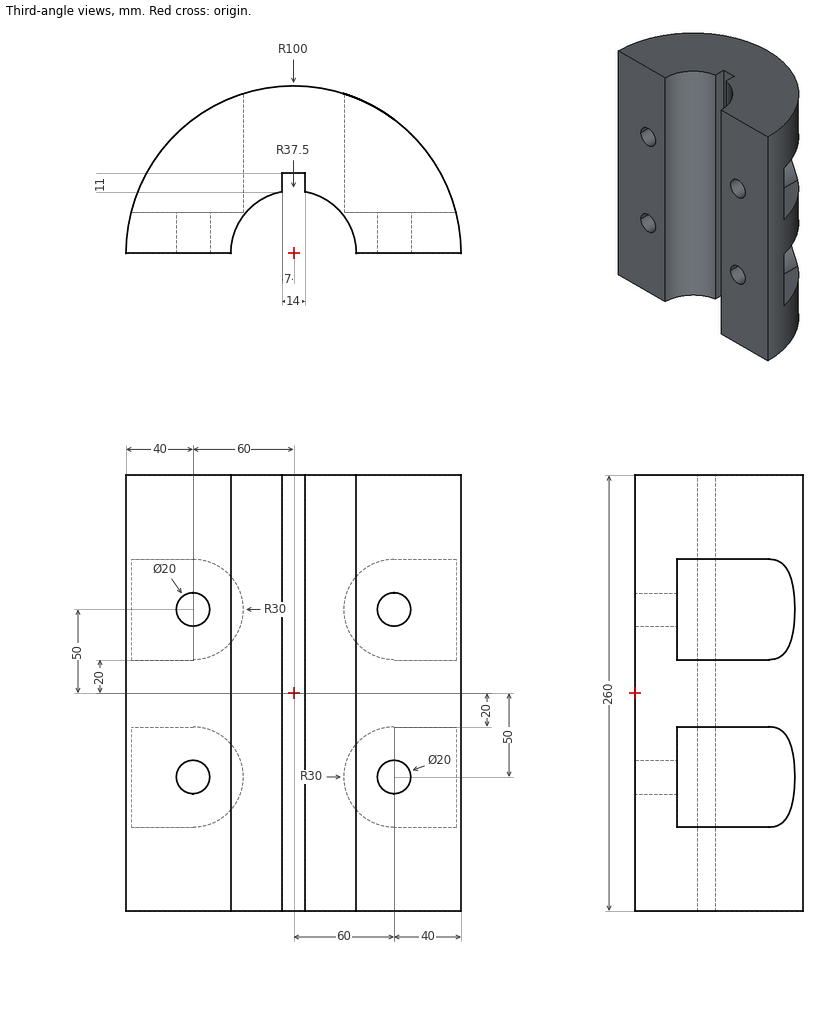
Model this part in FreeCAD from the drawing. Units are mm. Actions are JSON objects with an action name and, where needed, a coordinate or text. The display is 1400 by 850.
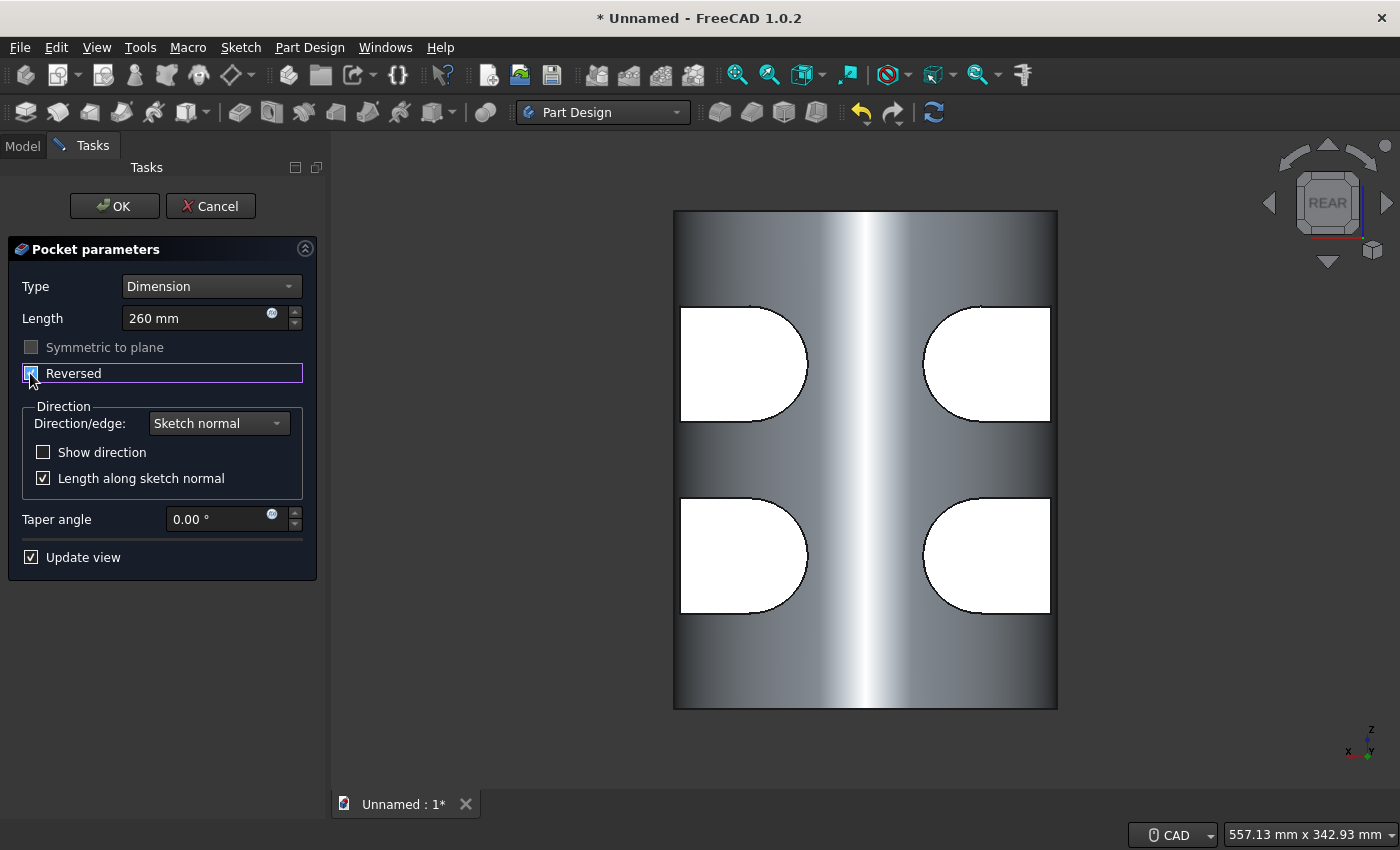
{"action": "left_click", "coordinate": [115, 206]}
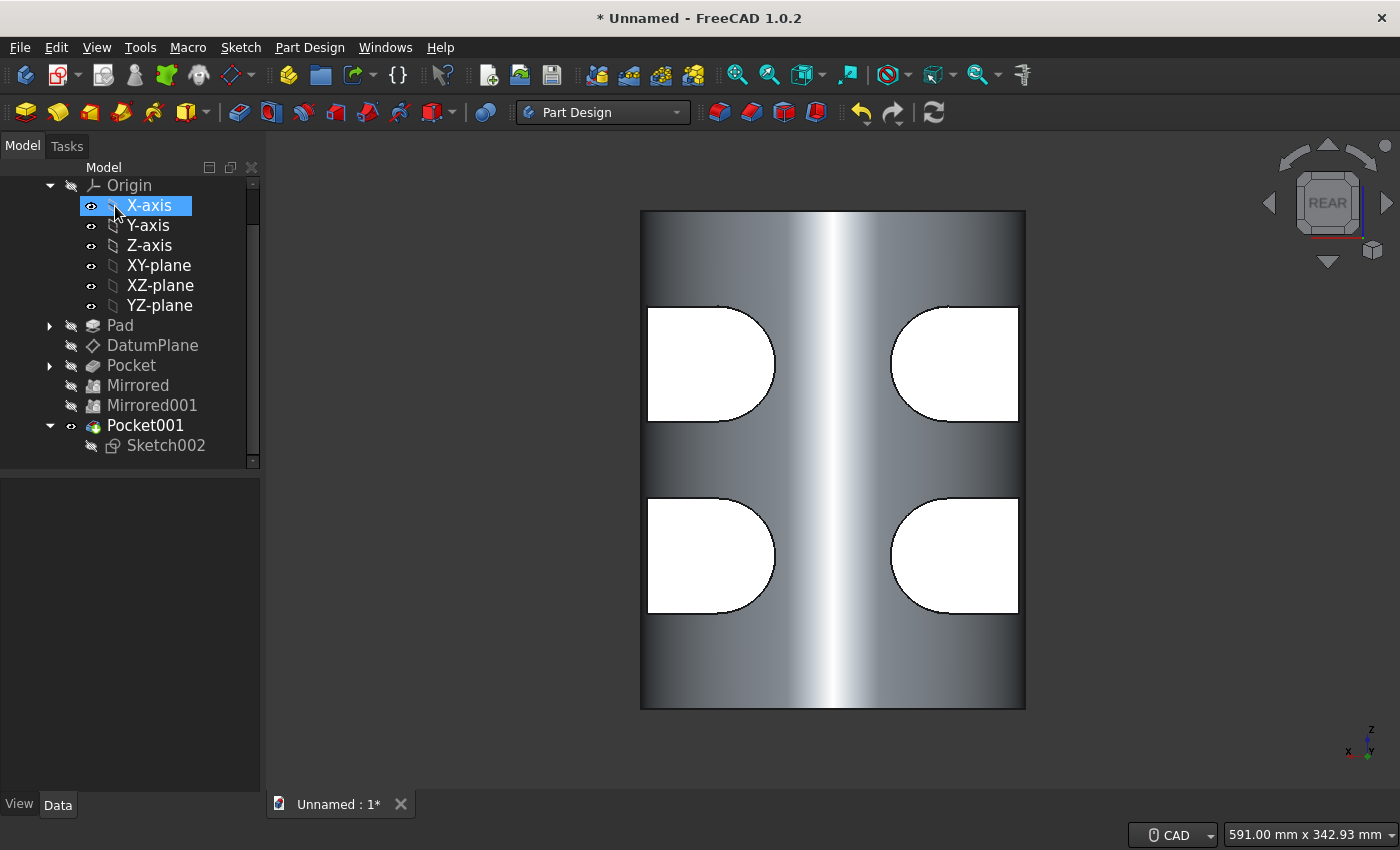
{"action": "left_click", "coordinate": [711, 363]}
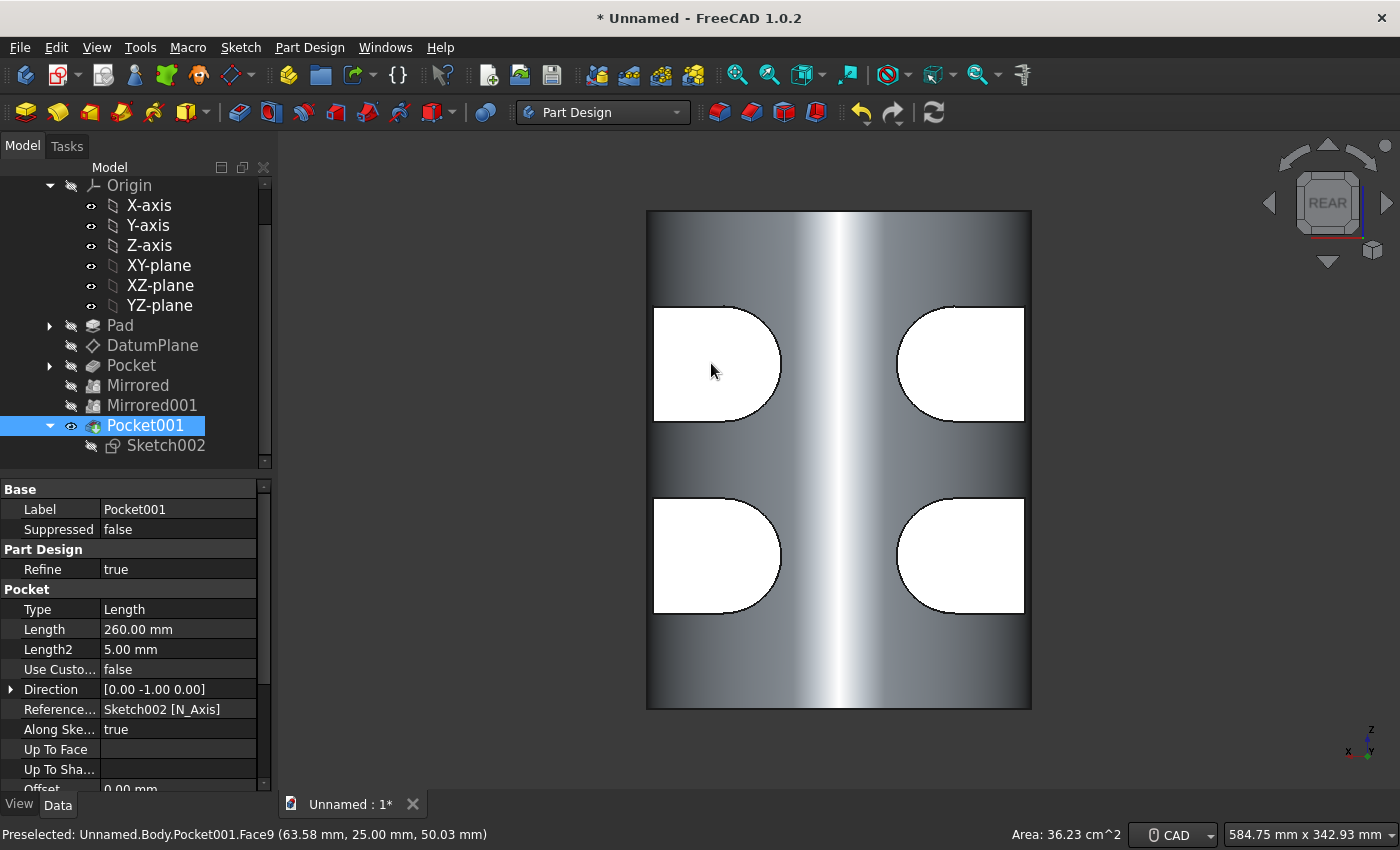
{"action": "left_click", "coordinate": [58, 76]}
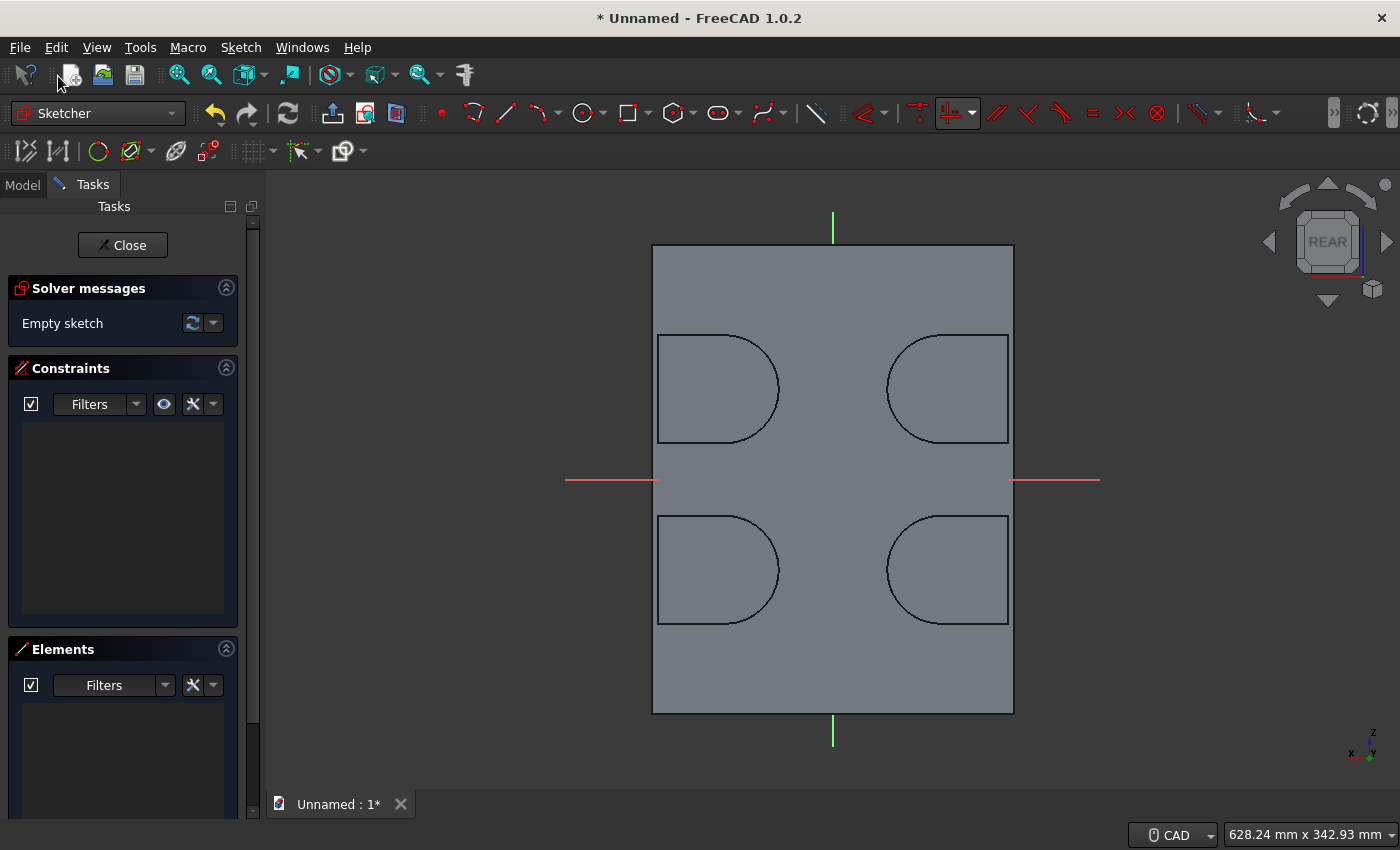
{"action": "left_click", "coordinate": [398, 114]}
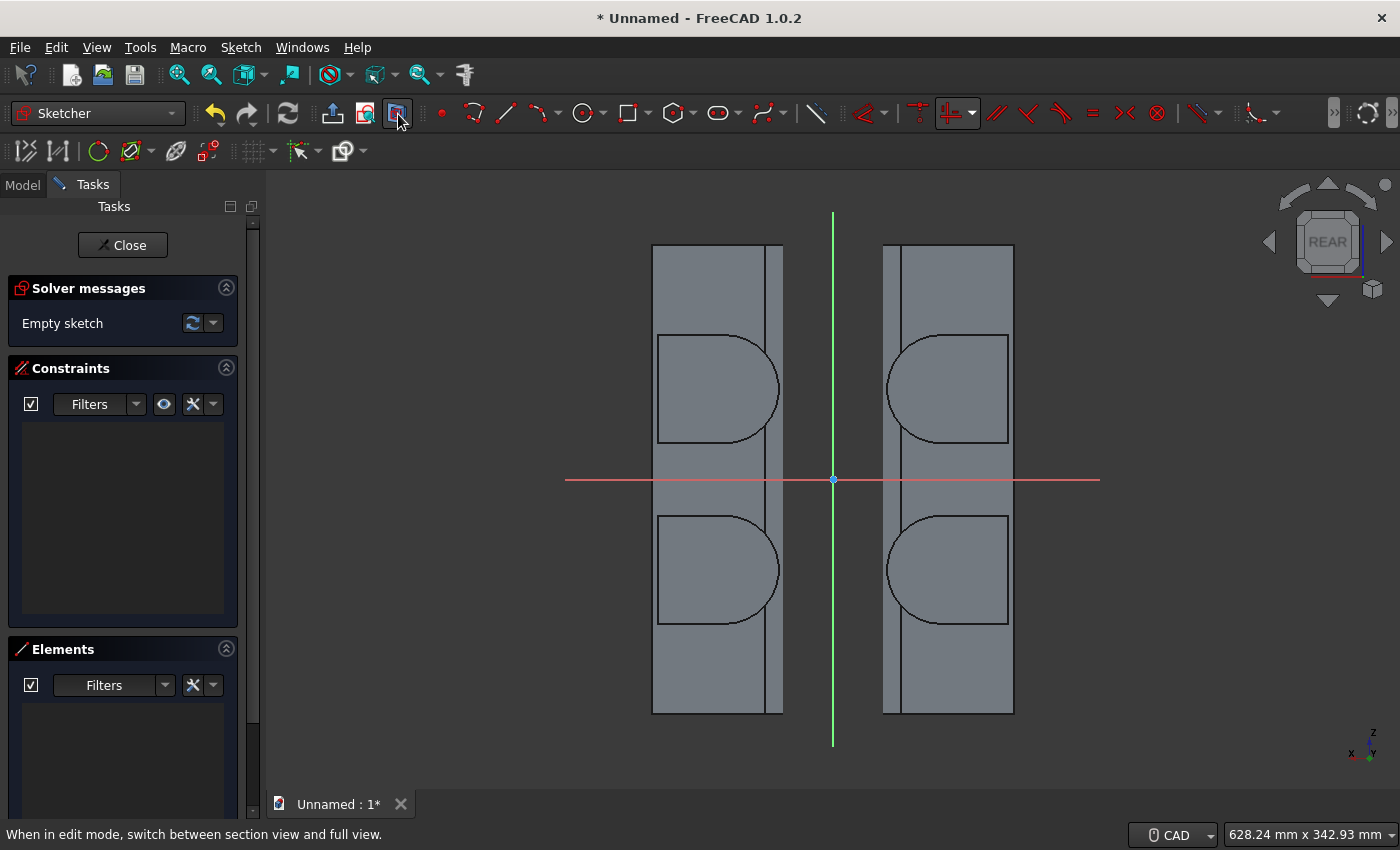
{"action": "scroll", "coordinate": [959, 380], "scroll_direction": "up", "scroll_amount": 12}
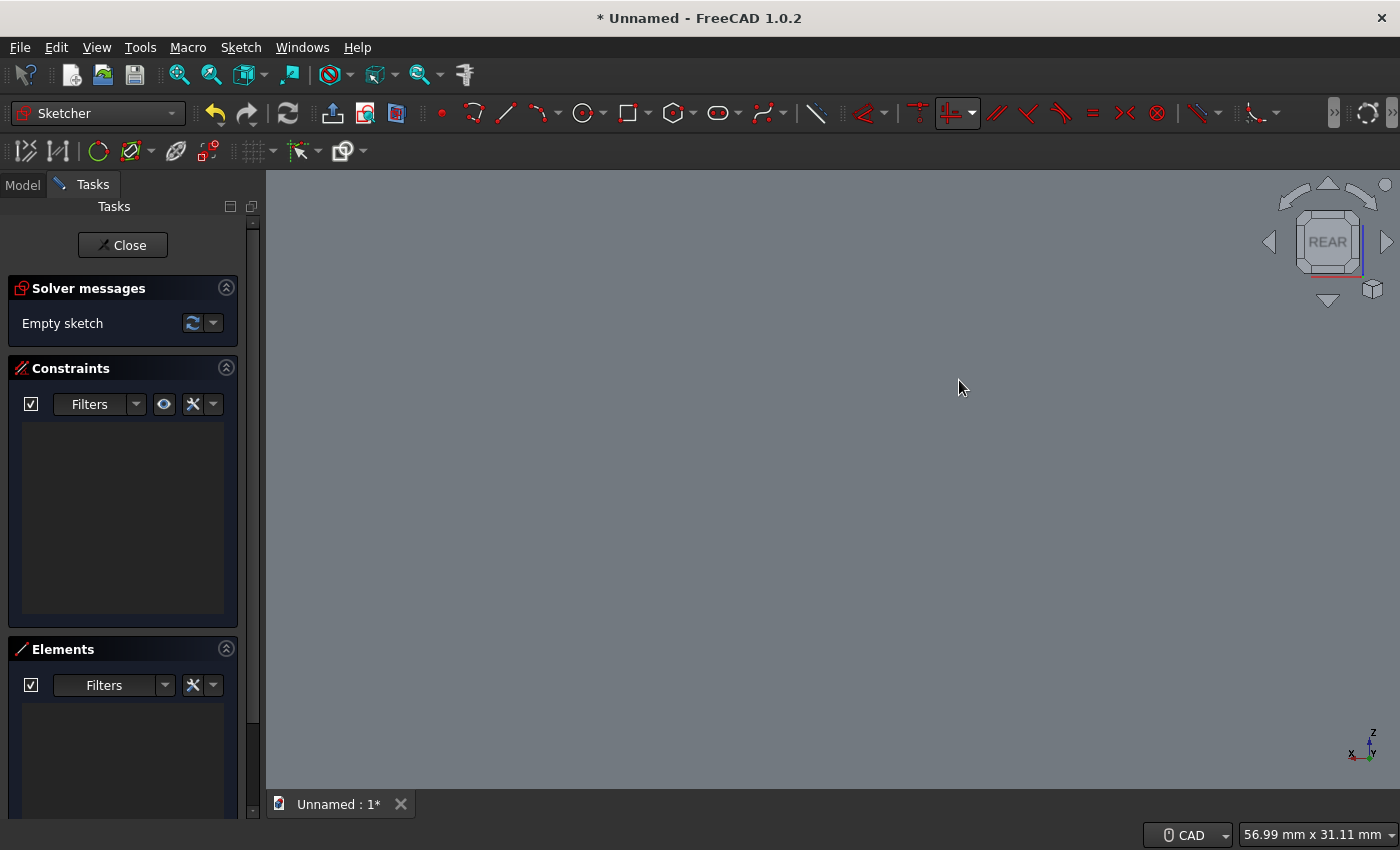
{"action": "left_click", "coordinate": [584, 114]}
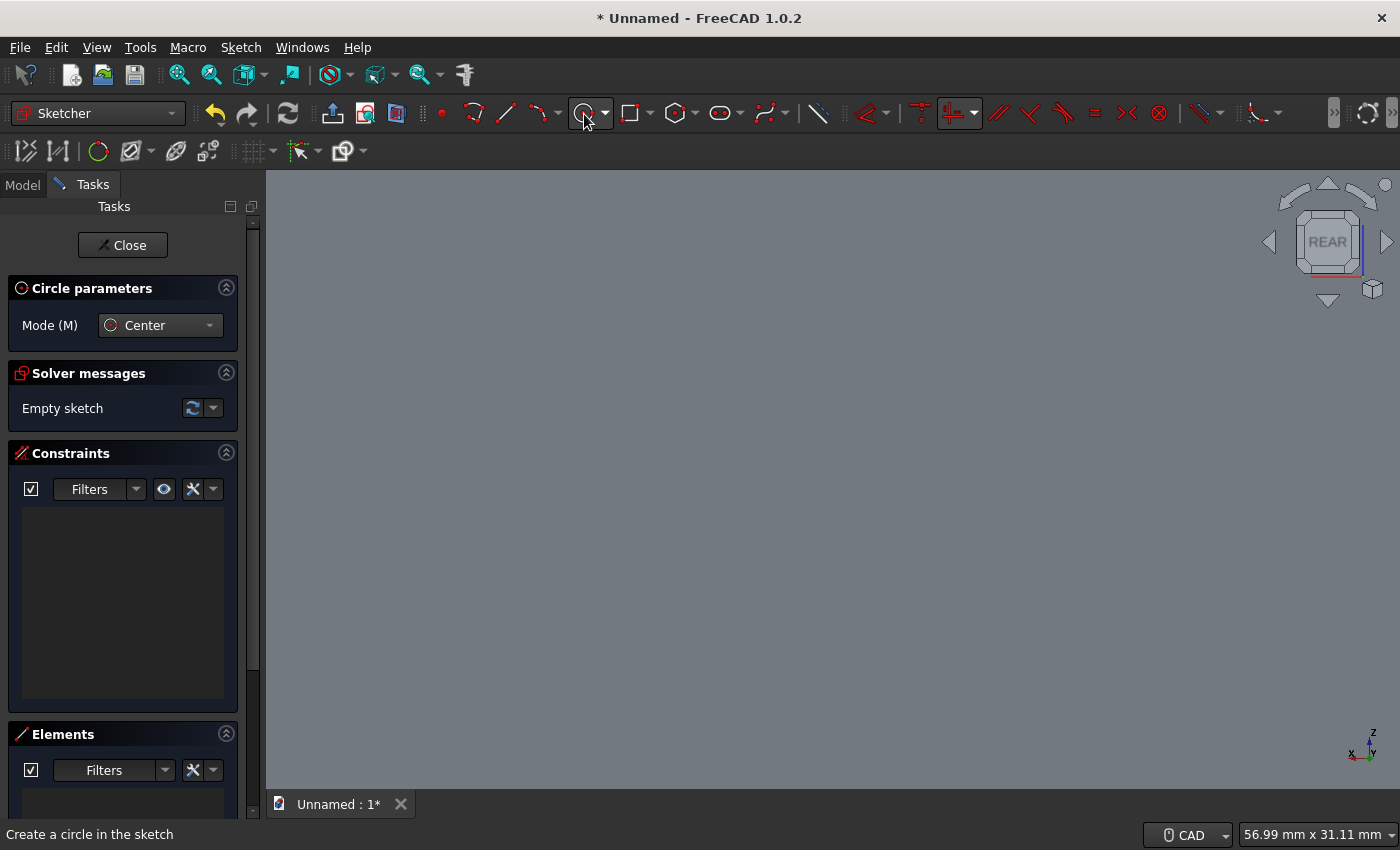
{"action": "left_click", "coordinate": [758, 479]}
{"action": "left_click", "coordinate": [898, 338]}
{"action": "key", "text": "Escape"}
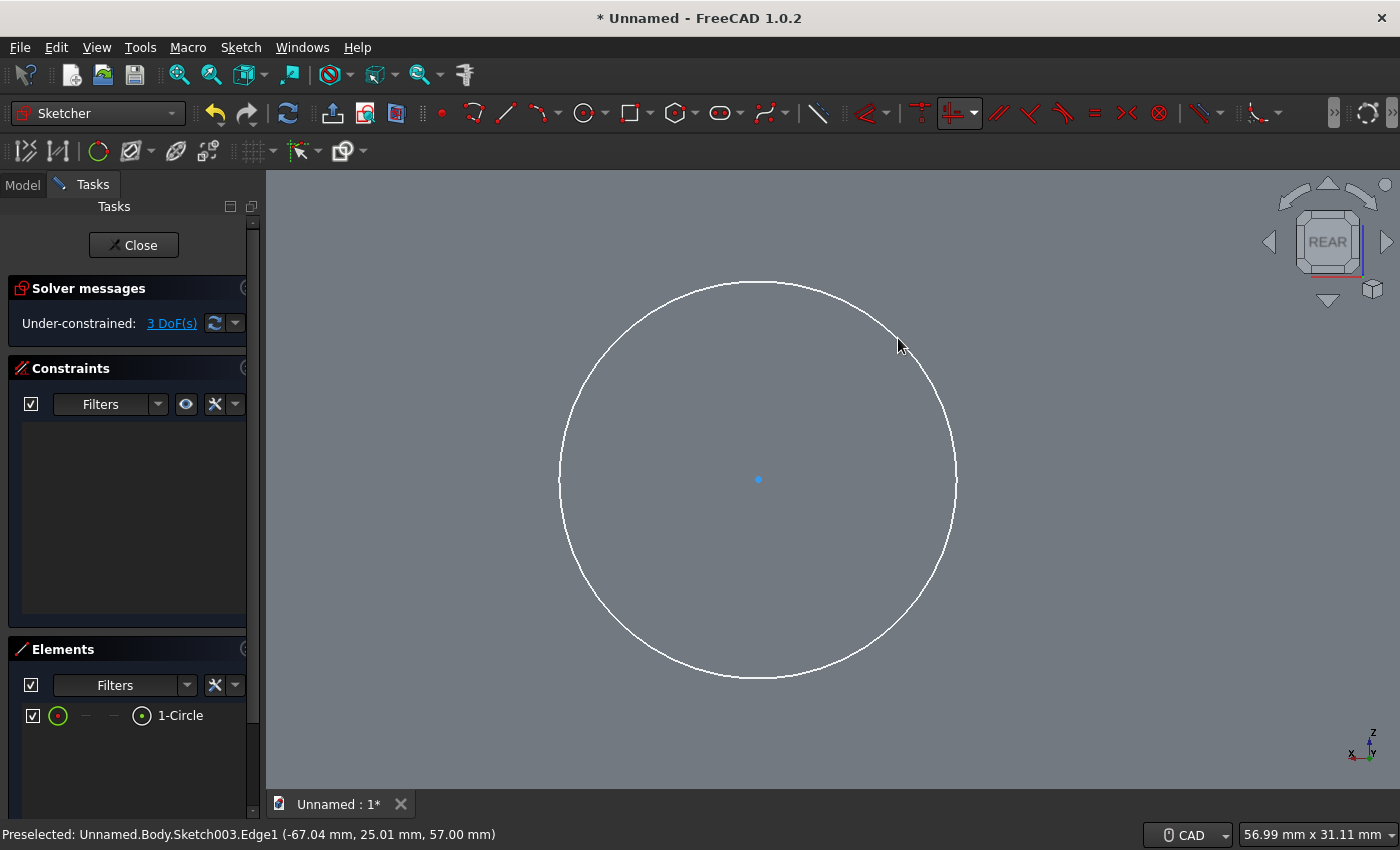
{"action": "left_click", "coordinate": [866, 114]}